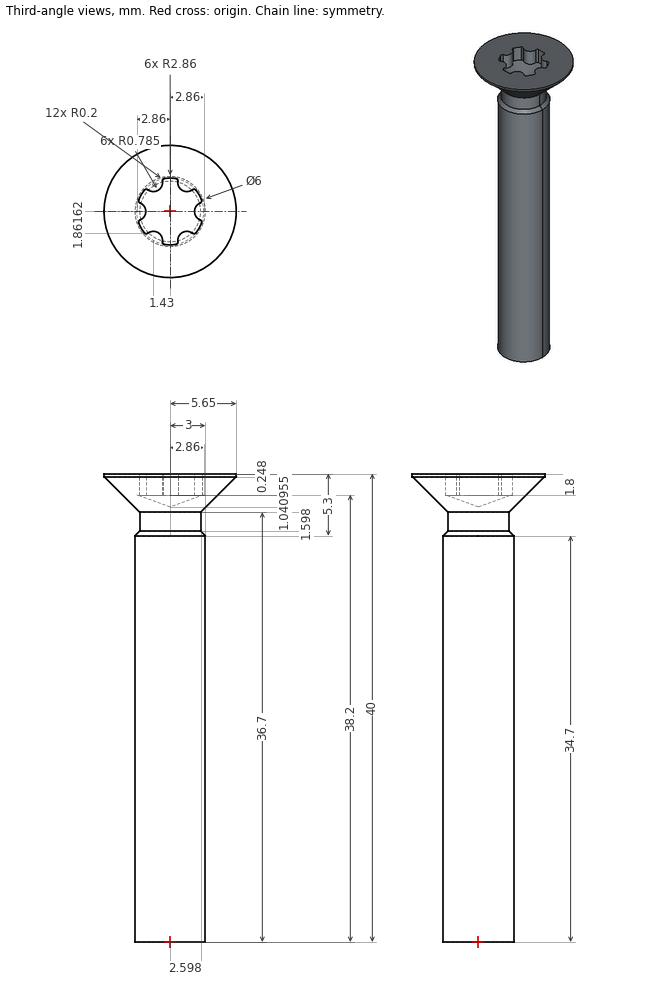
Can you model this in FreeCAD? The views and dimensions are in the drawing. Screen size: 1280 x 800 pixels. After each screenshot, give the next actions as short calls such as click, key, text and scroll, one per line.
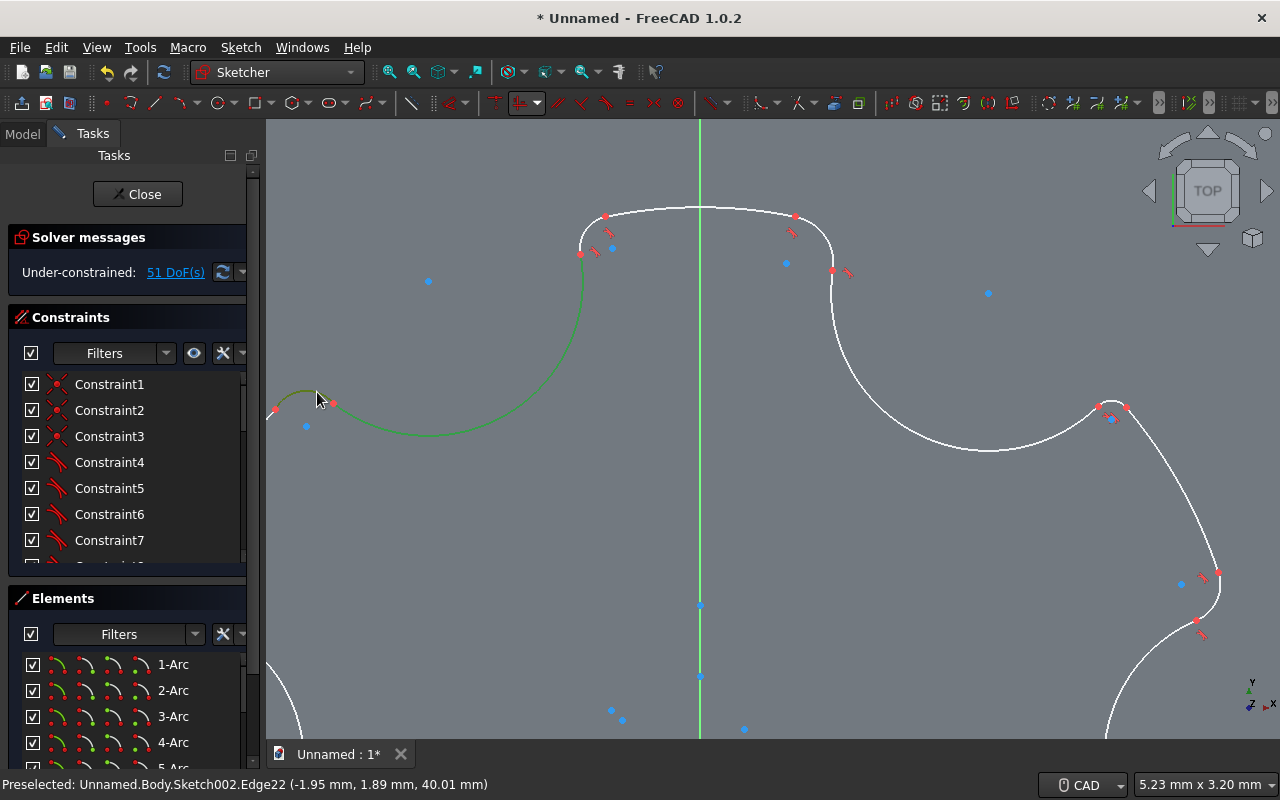
click(606, 104)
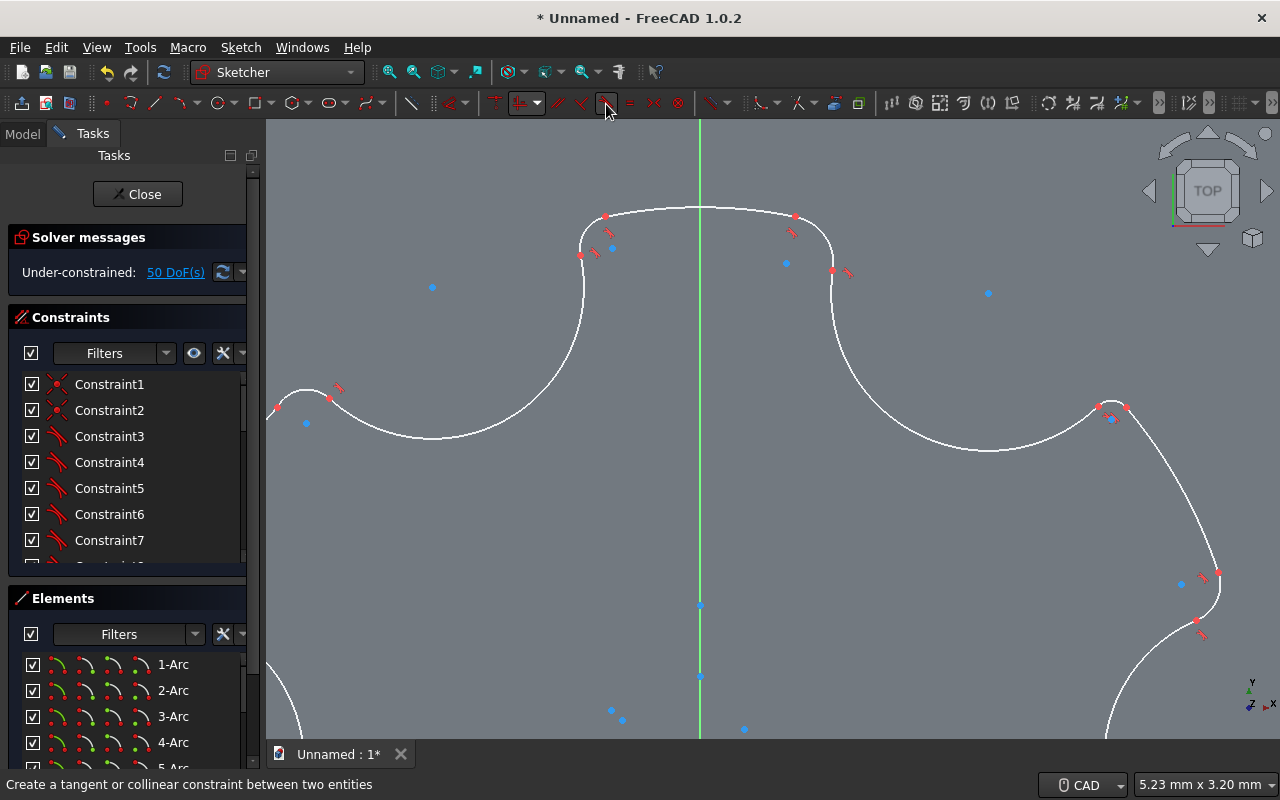
click(313, 390)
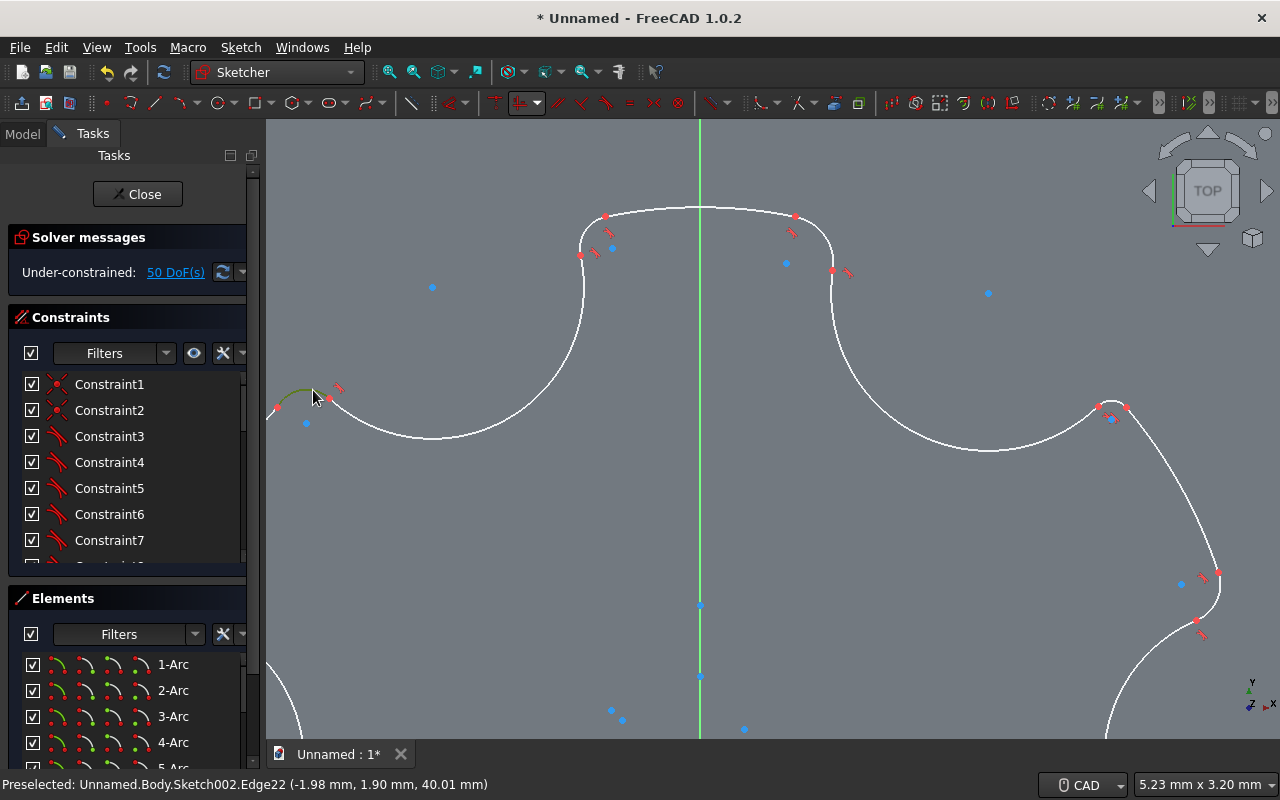
scroll(707, 236, down, 5)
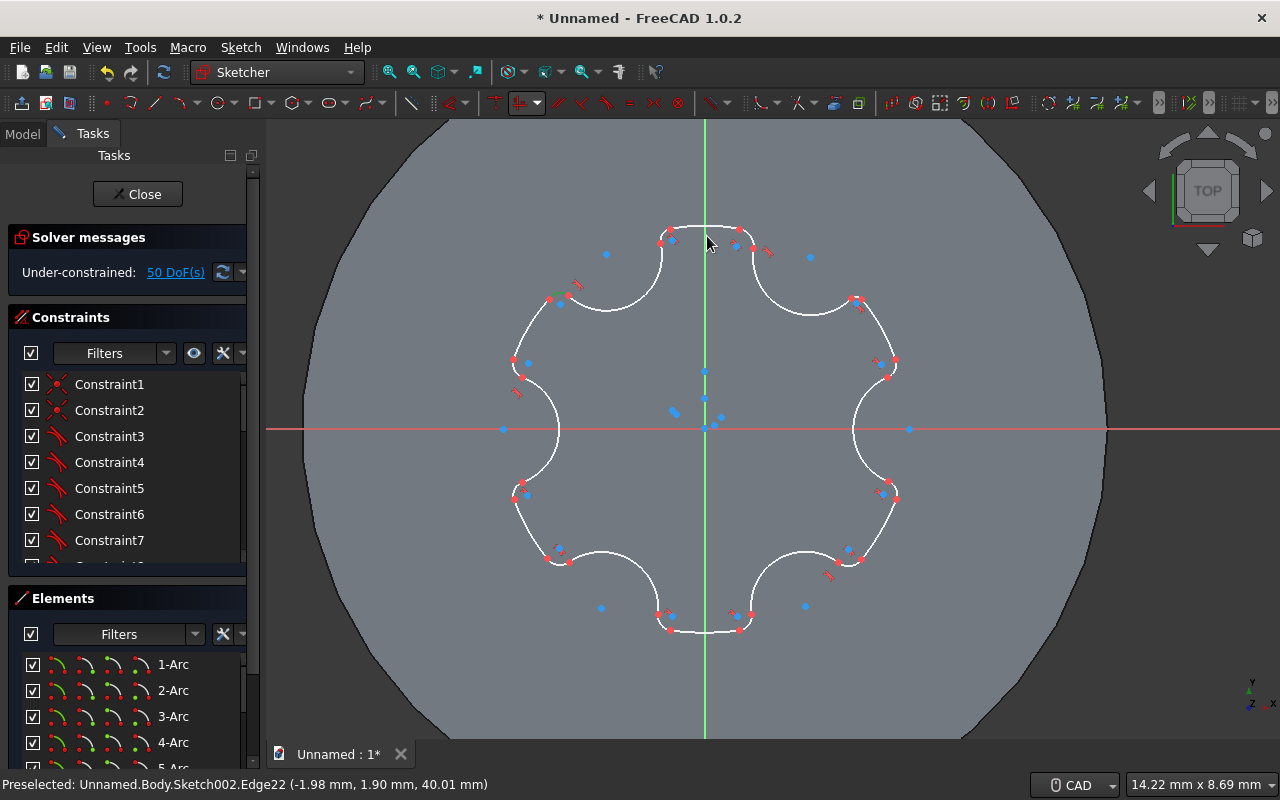
click(536, 315)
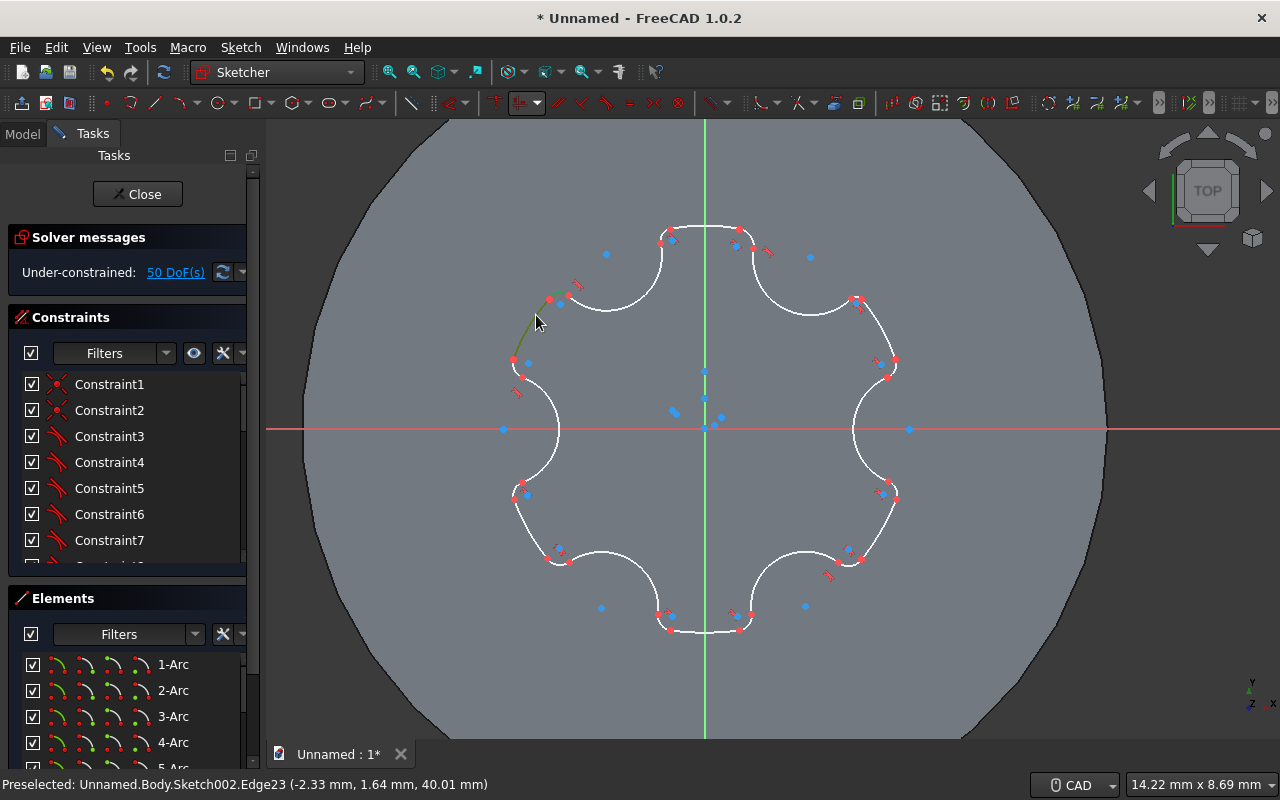
click(606, 104)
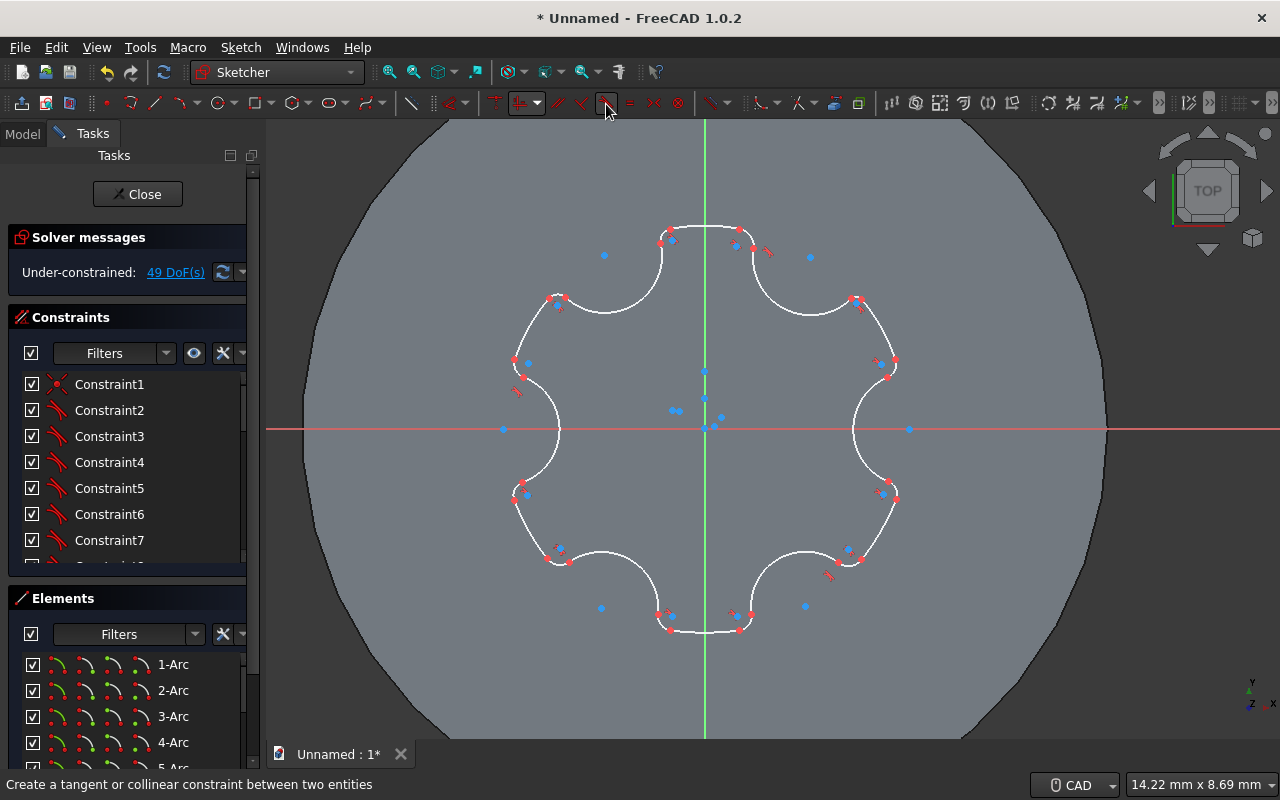
click(536, 315)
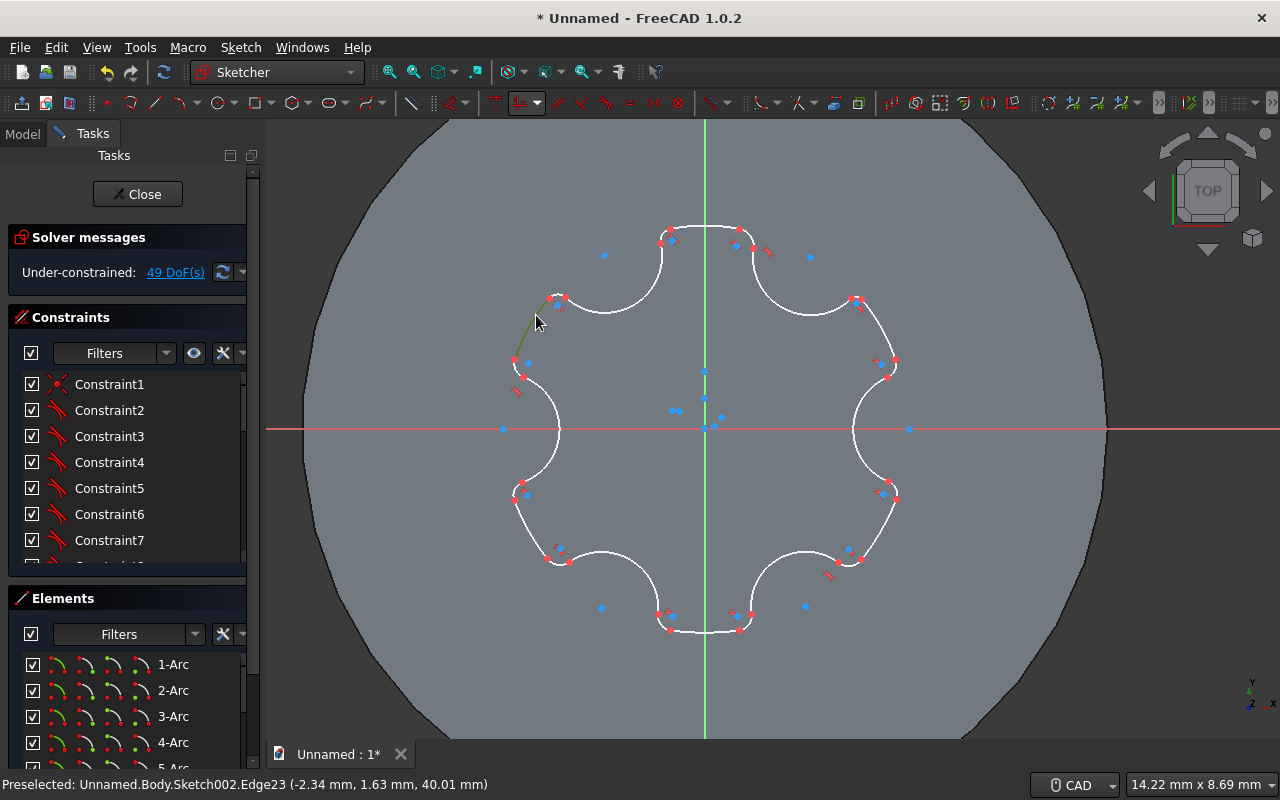
scroll(516, 370, up, 2)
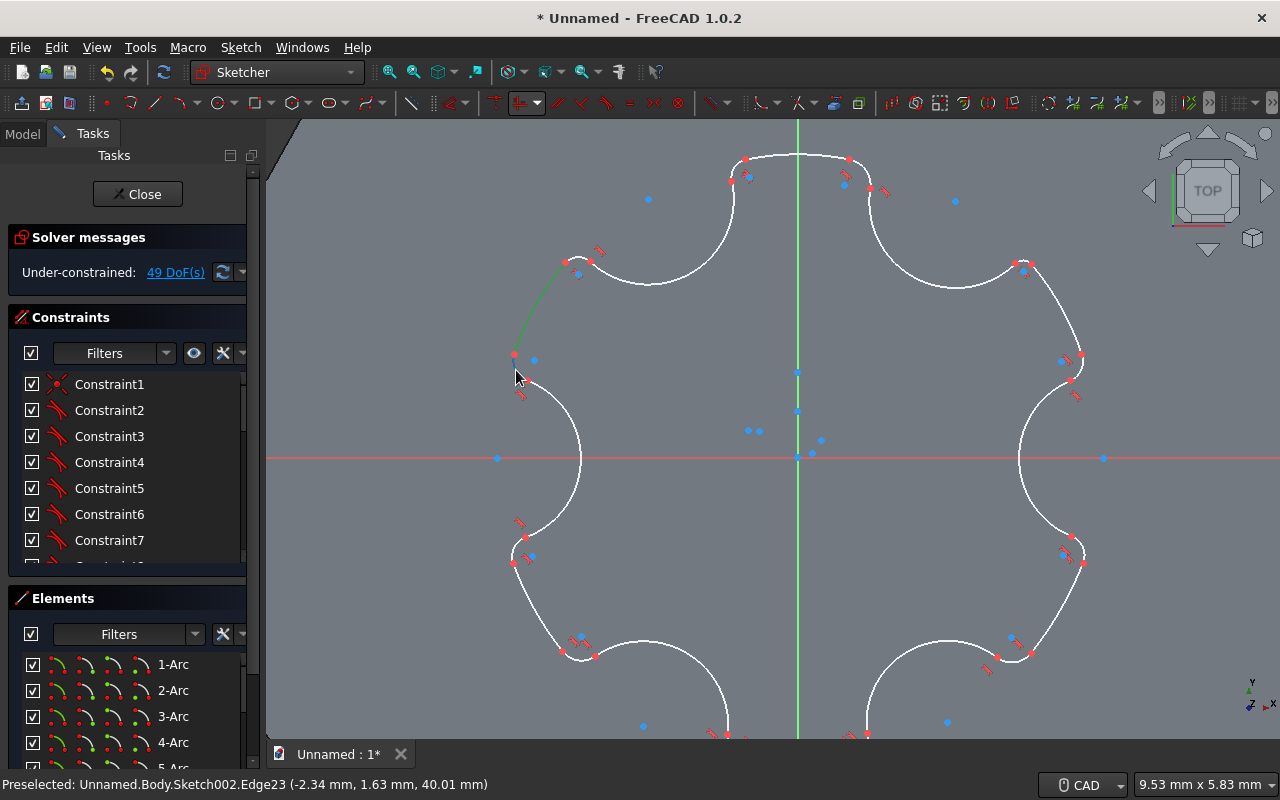
click(516, 370)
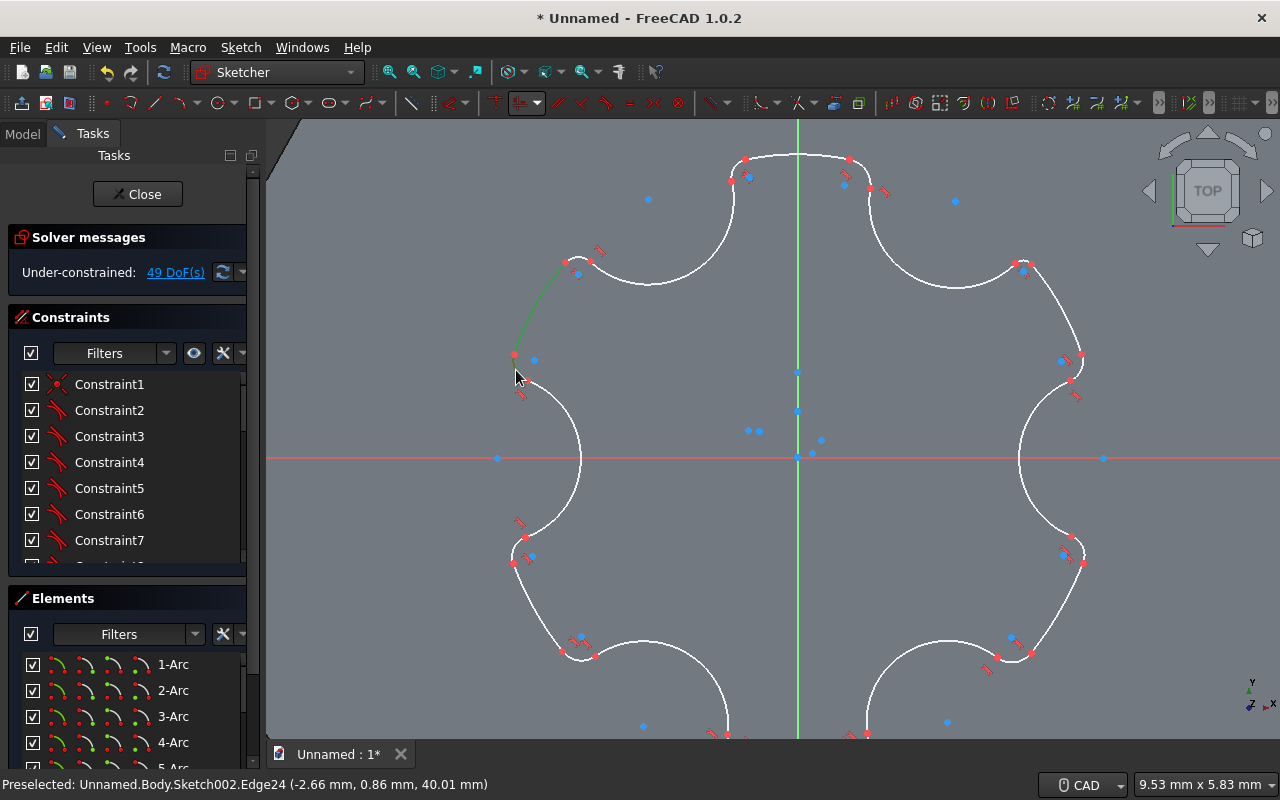
key(t)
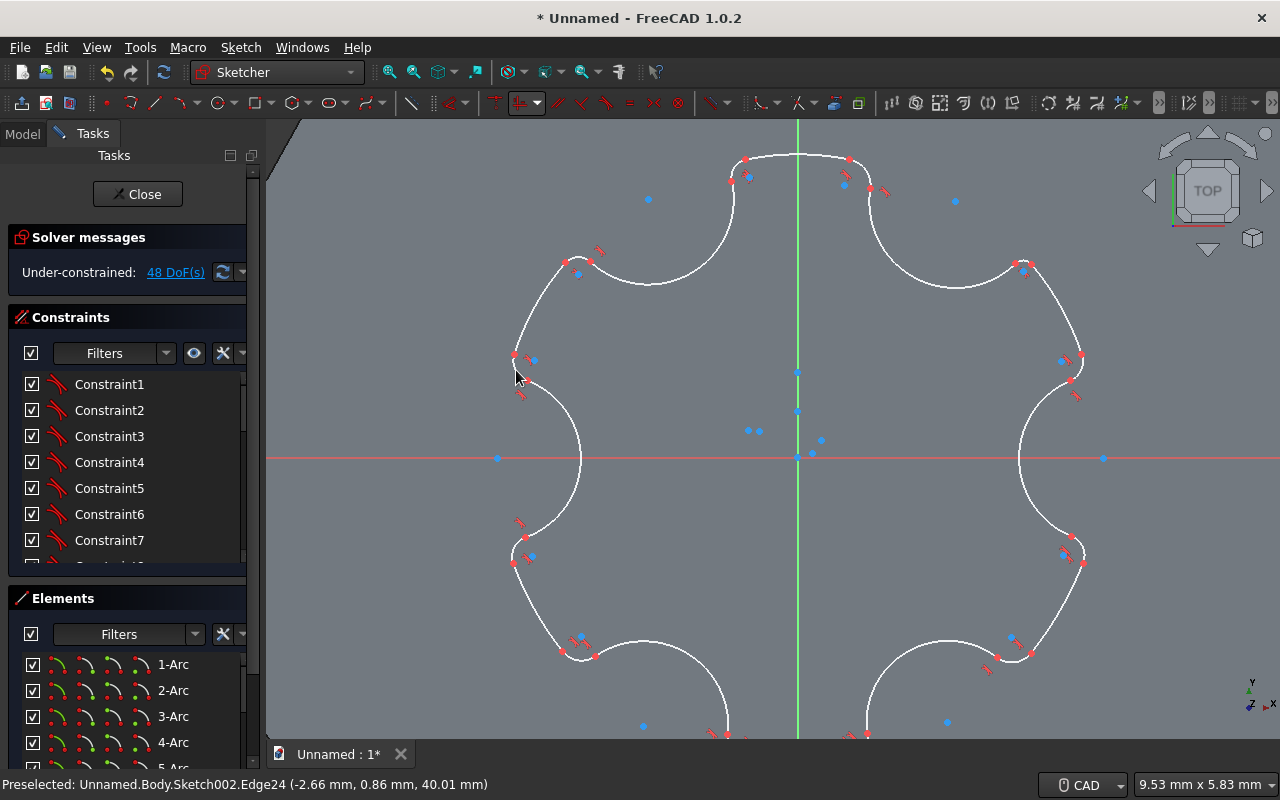
click(525, 592)